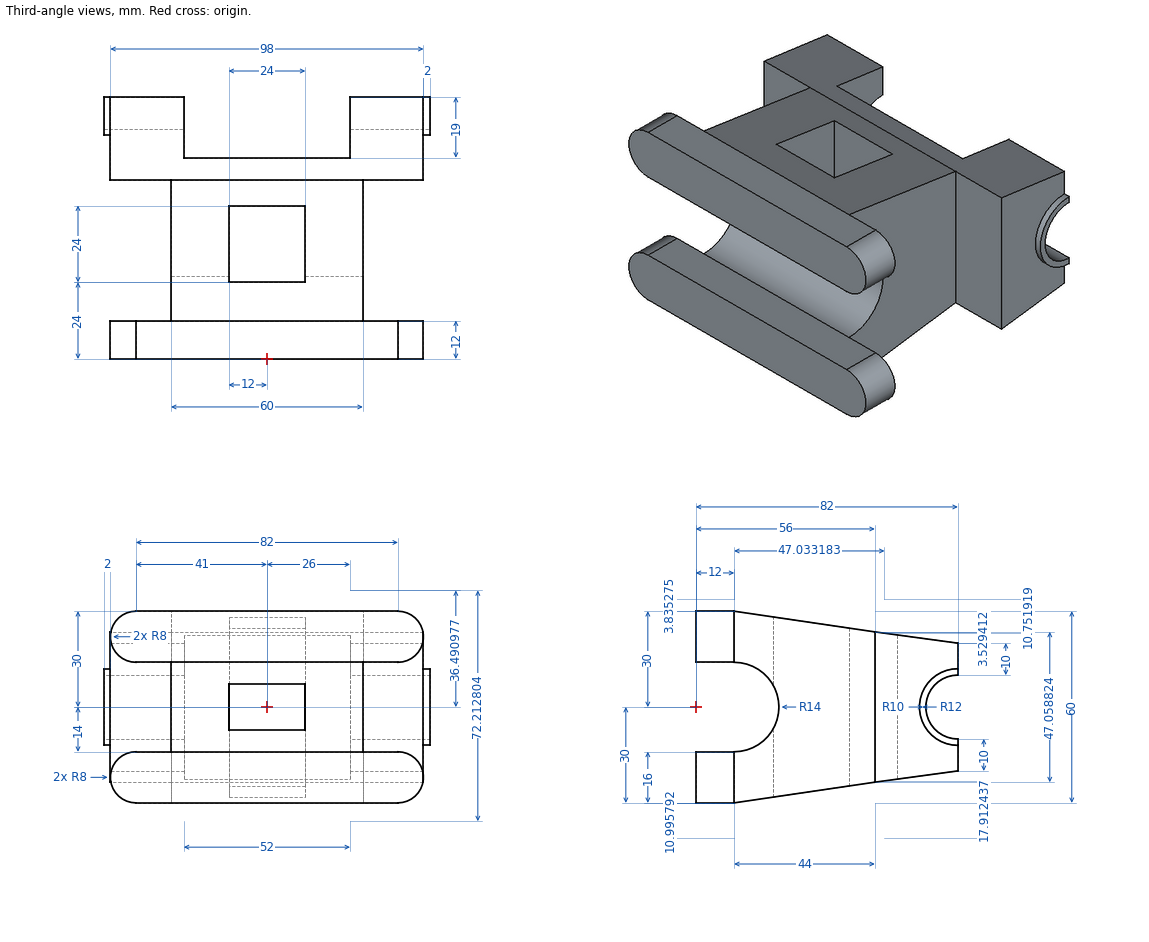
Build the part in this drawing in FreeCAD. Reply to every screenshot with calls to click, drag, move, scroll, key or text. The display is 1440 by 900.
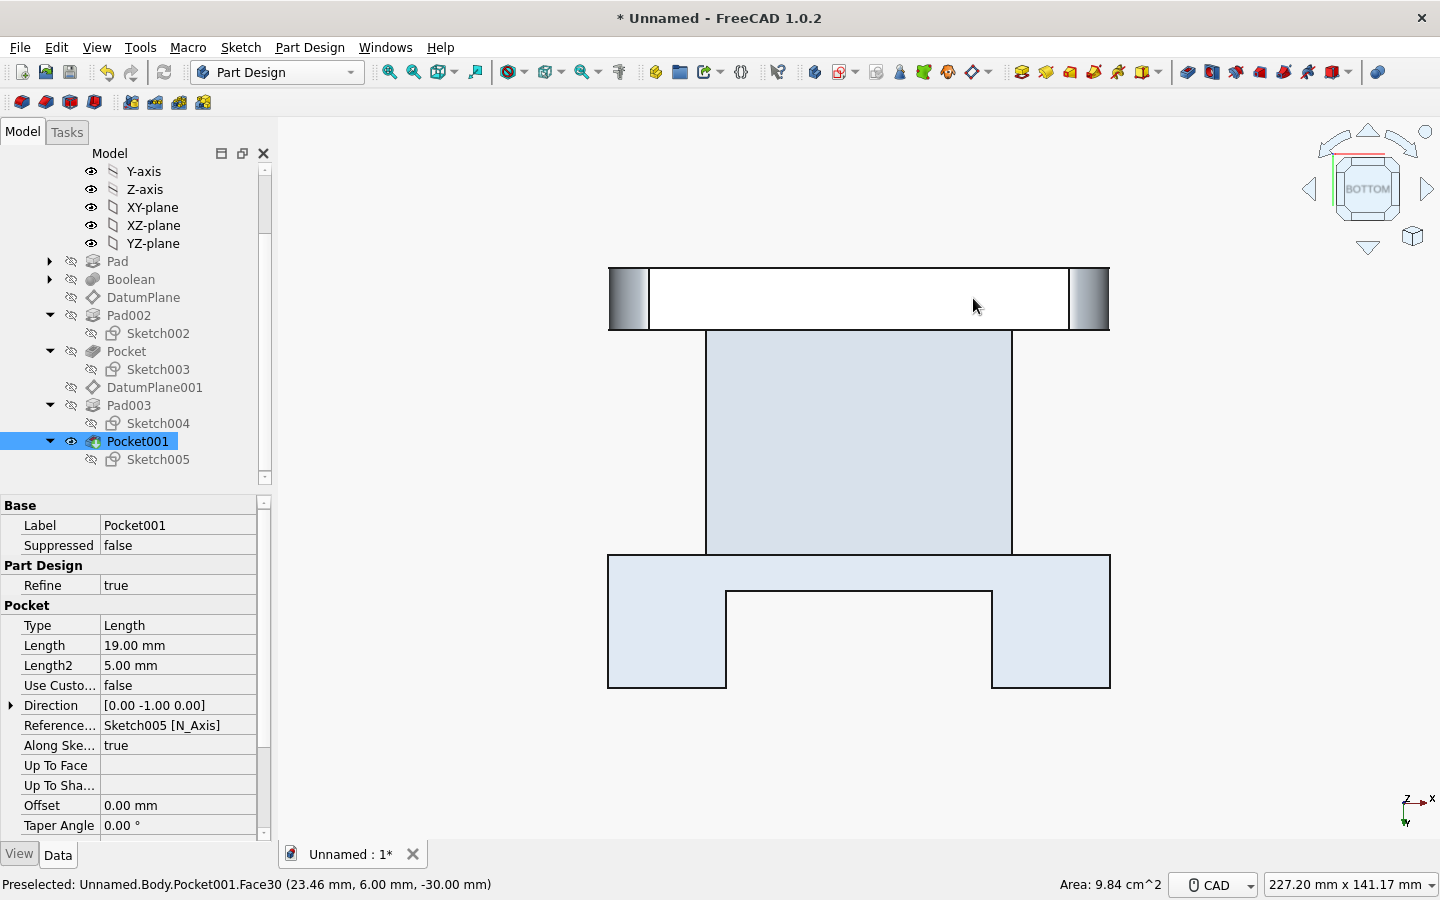
click(840, 72)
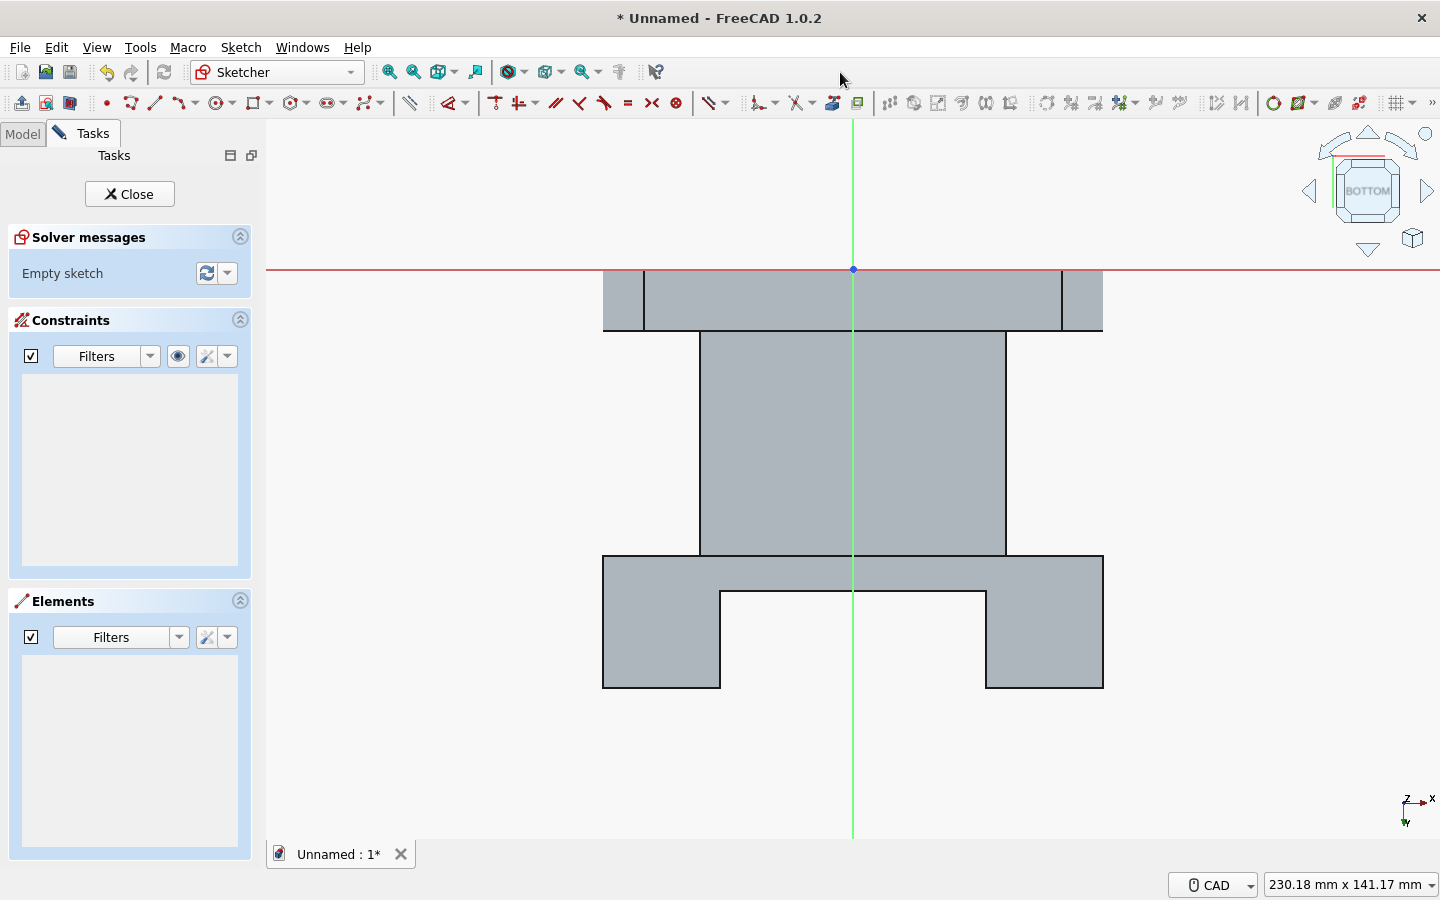
scroll(936, 287, up, 3)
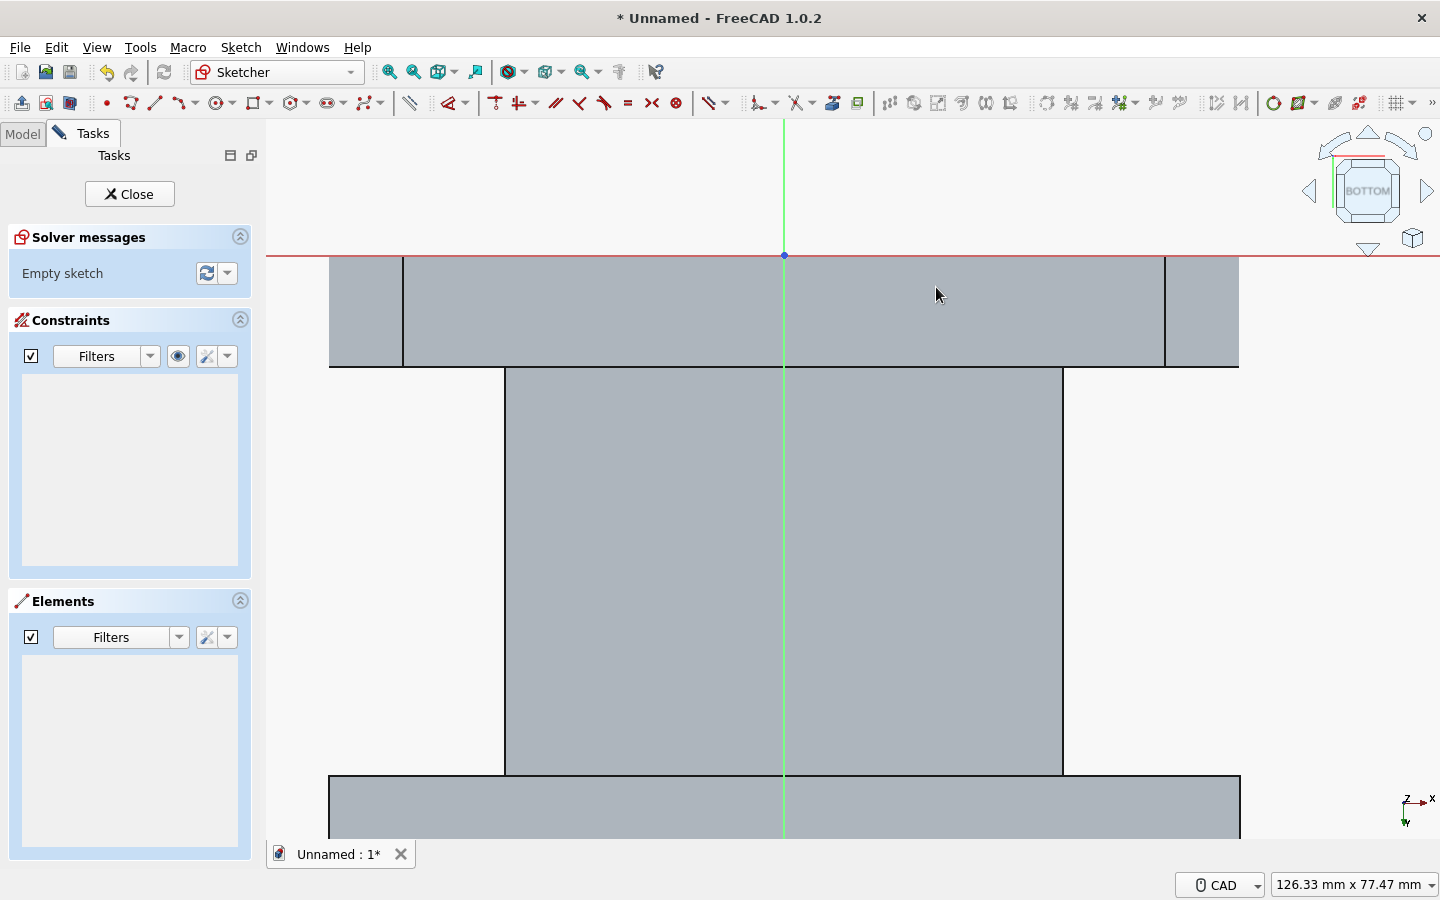
click(254, 104)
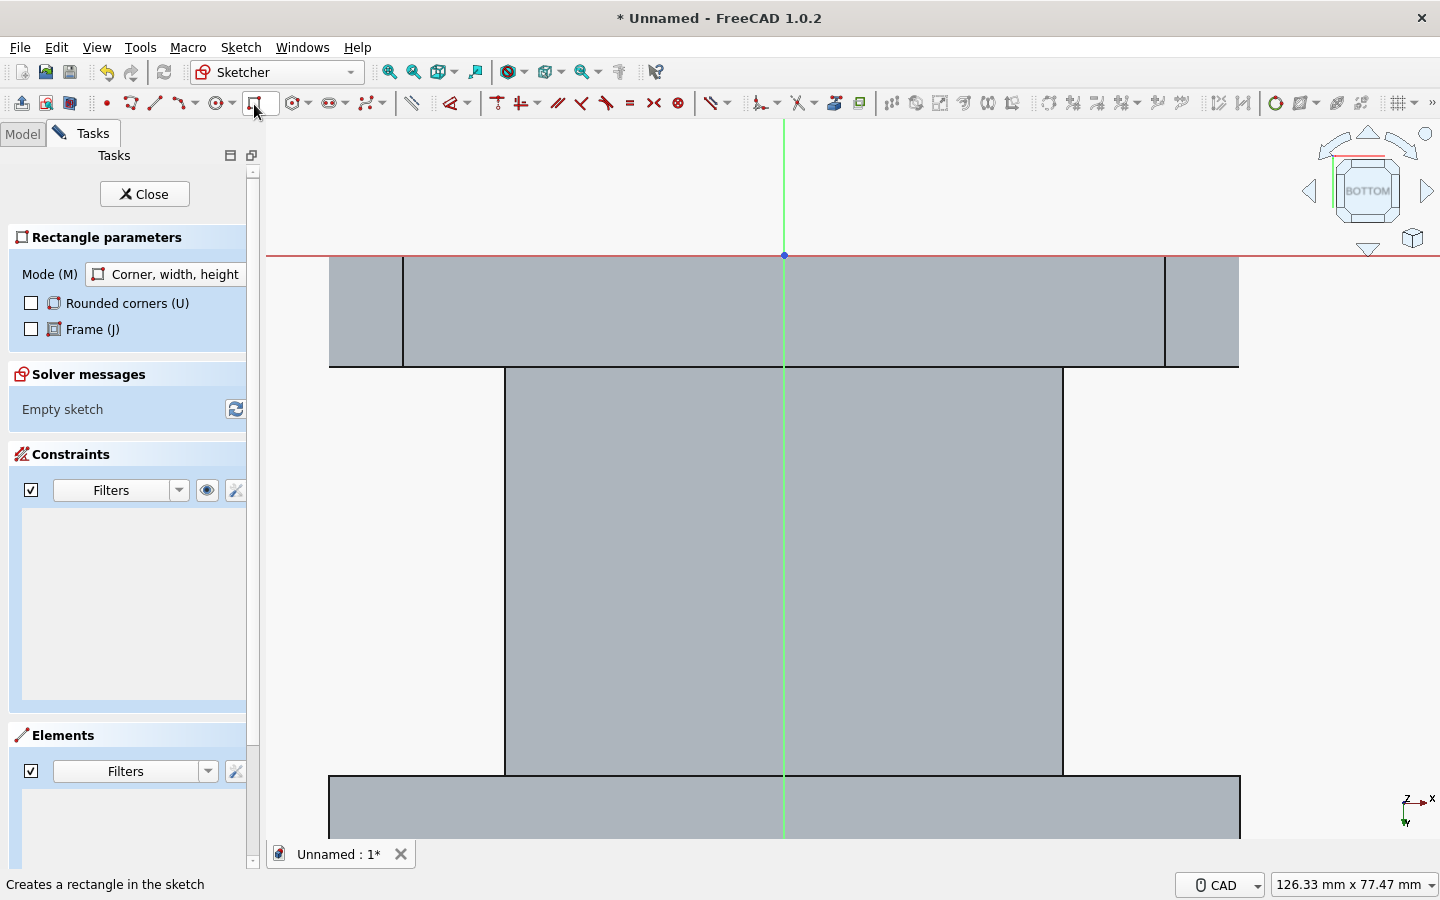
click(673, 479)
click(896, 702)
key(Escape)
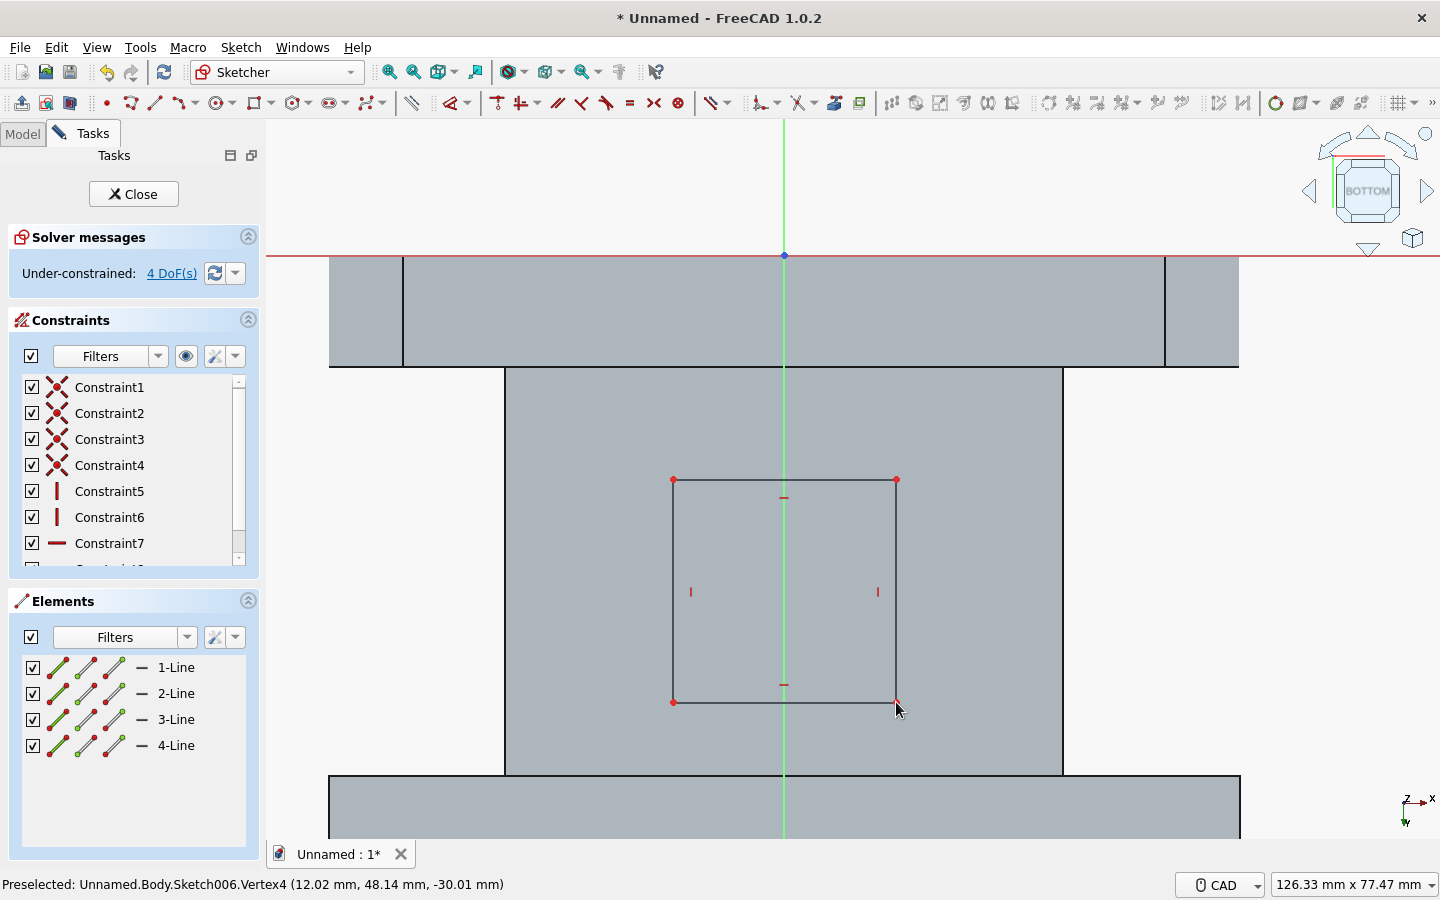
click(450, 104)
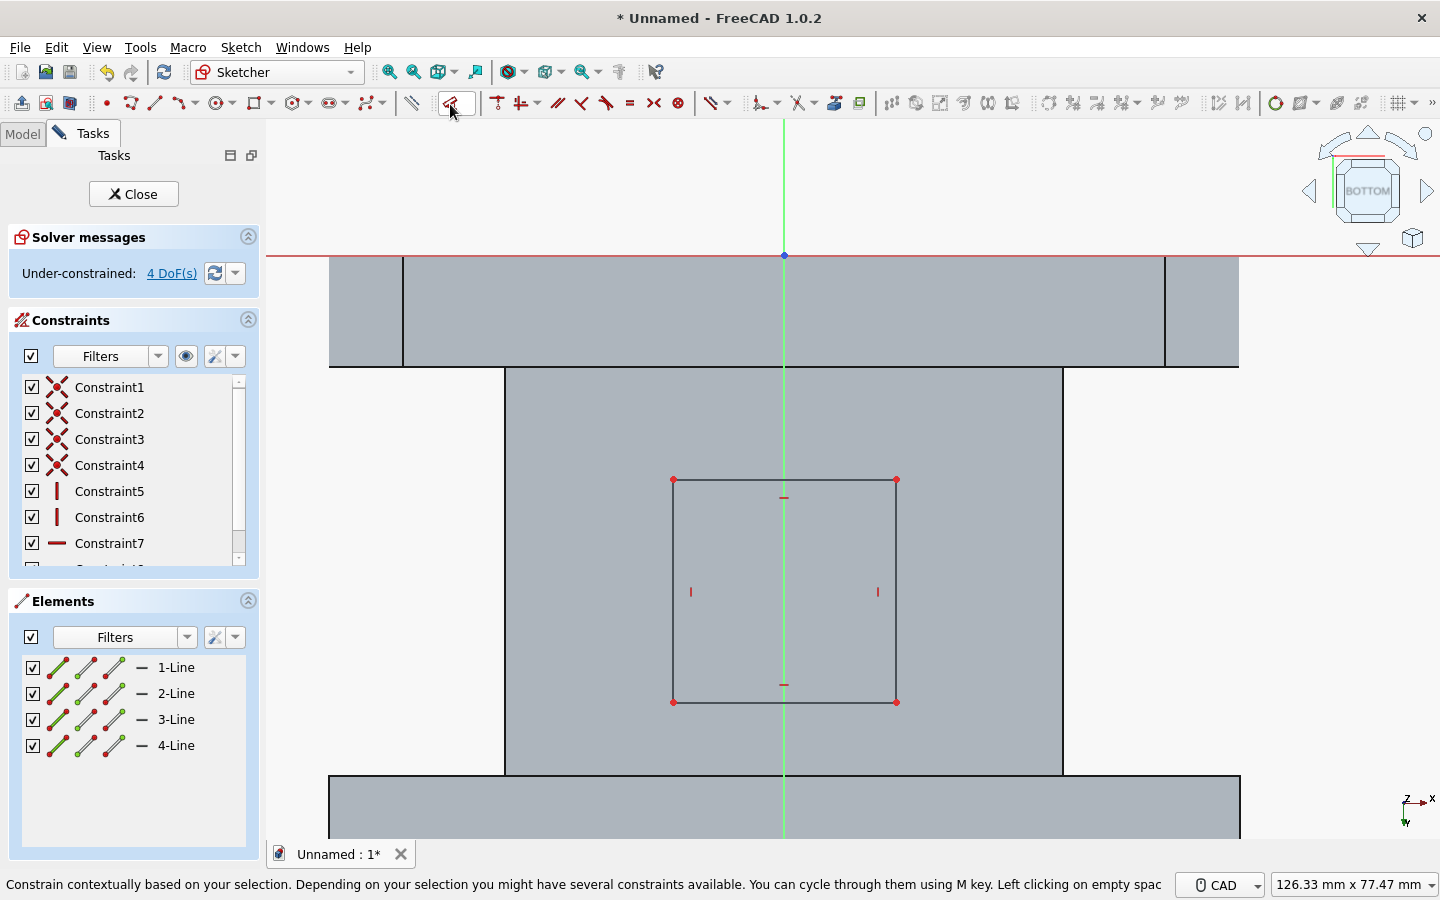
click(673, 547)
click(639, 591)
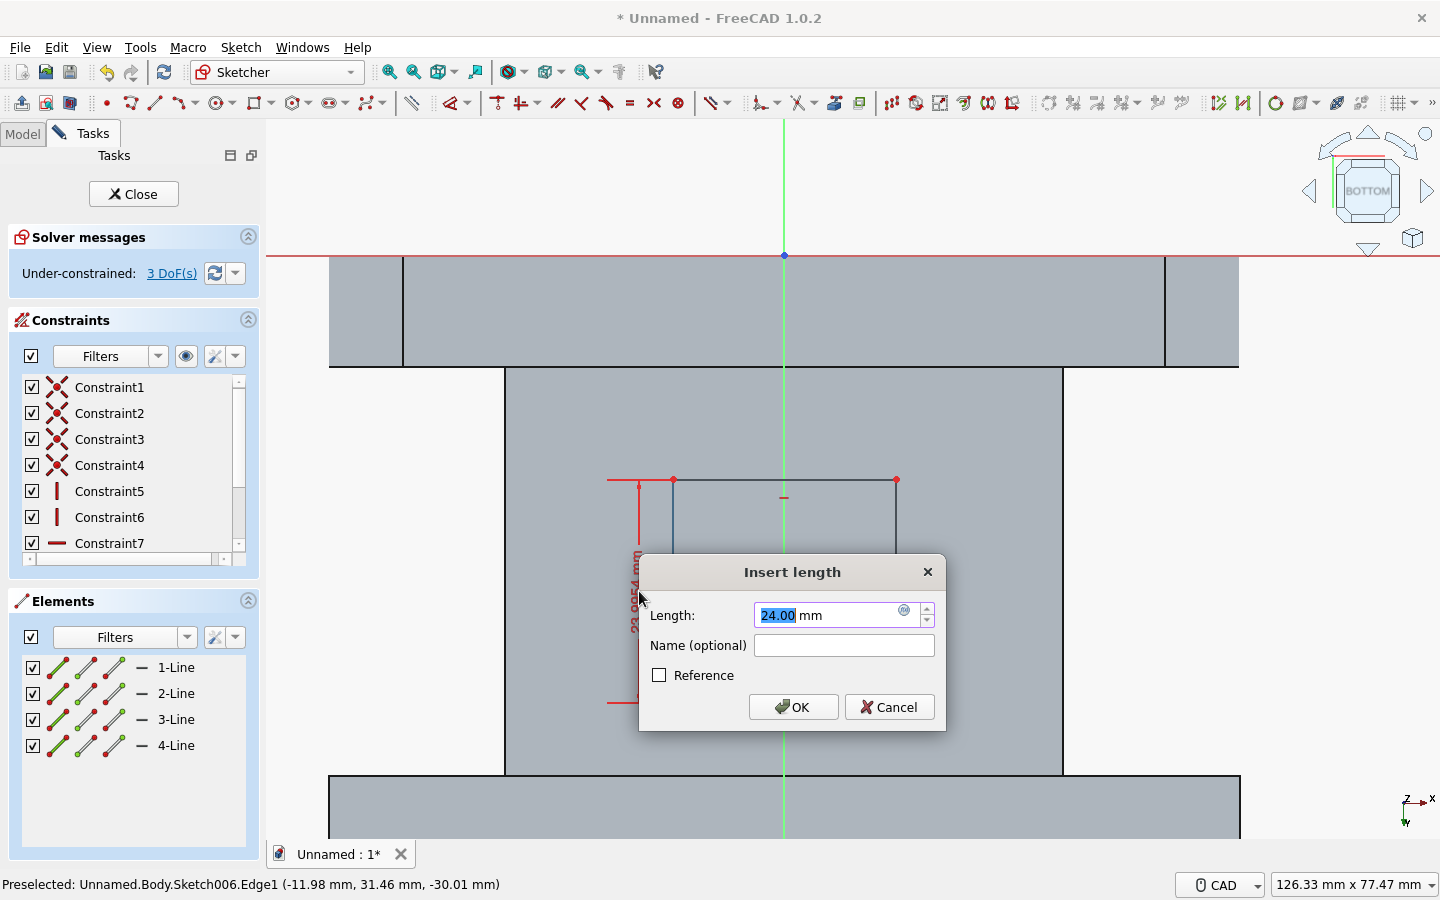
text(24)
key(Return)